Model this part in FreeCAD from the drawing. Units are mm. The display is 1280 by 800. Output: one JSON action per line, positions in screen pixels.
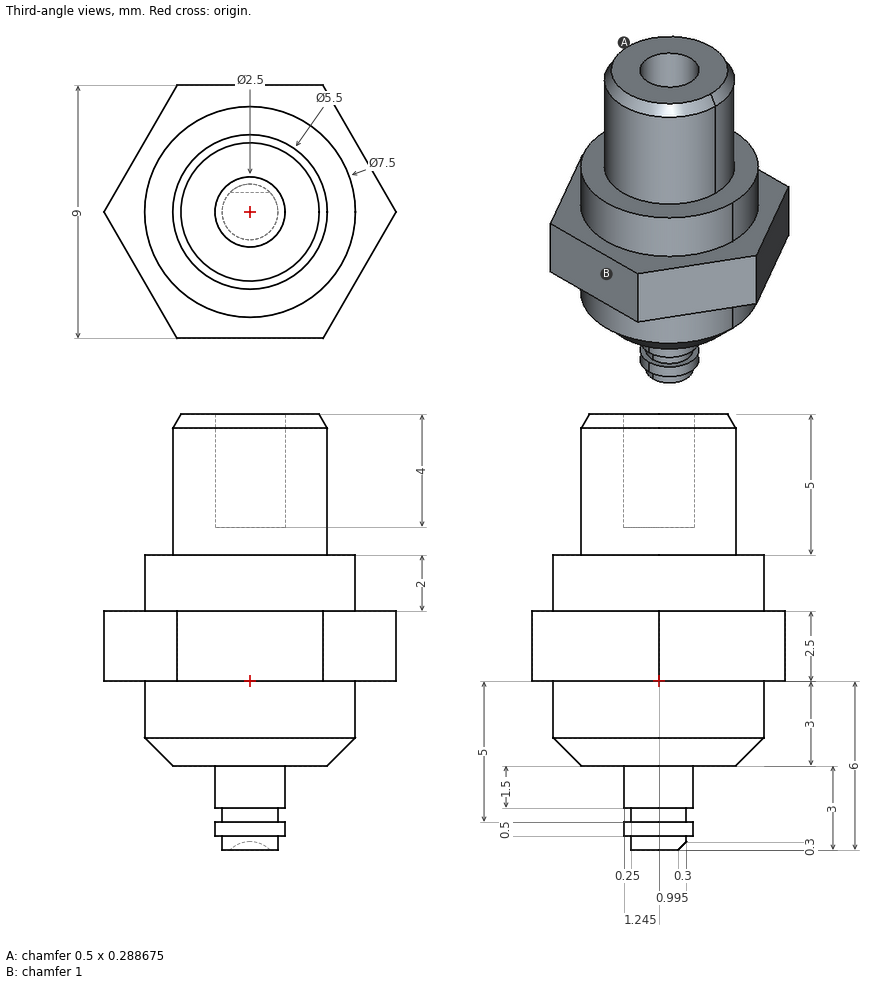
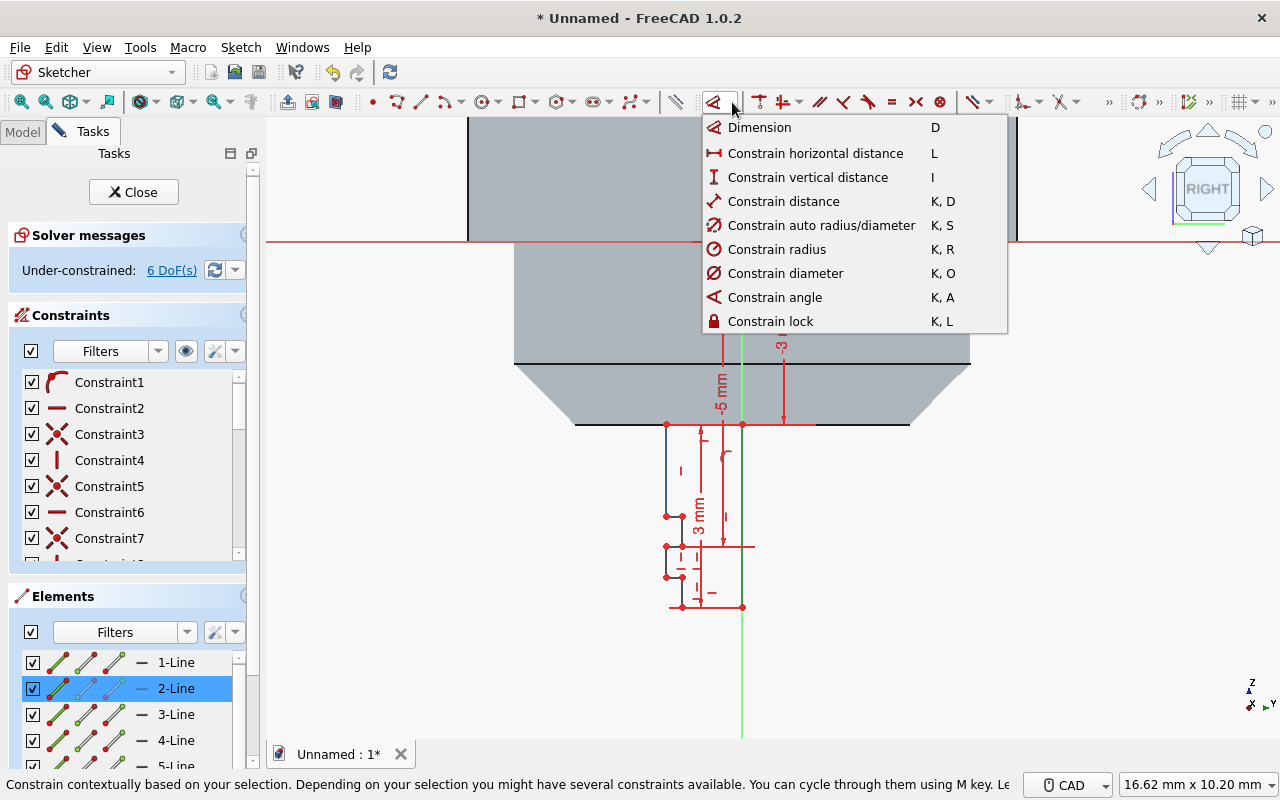
{"action": "left_click", "coordinate": [855, 177]}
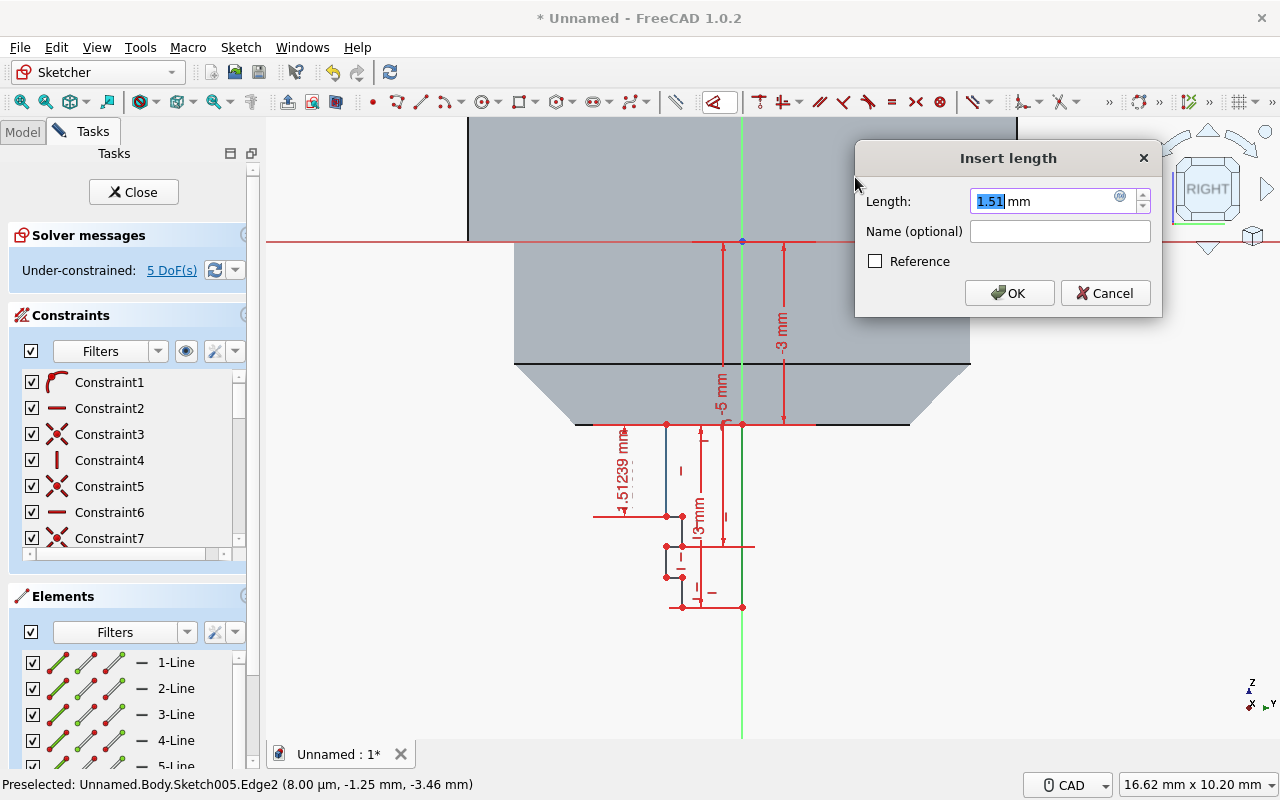
{"action": "type", "text": "1.5"}
{"action": "key", "text": "Return"}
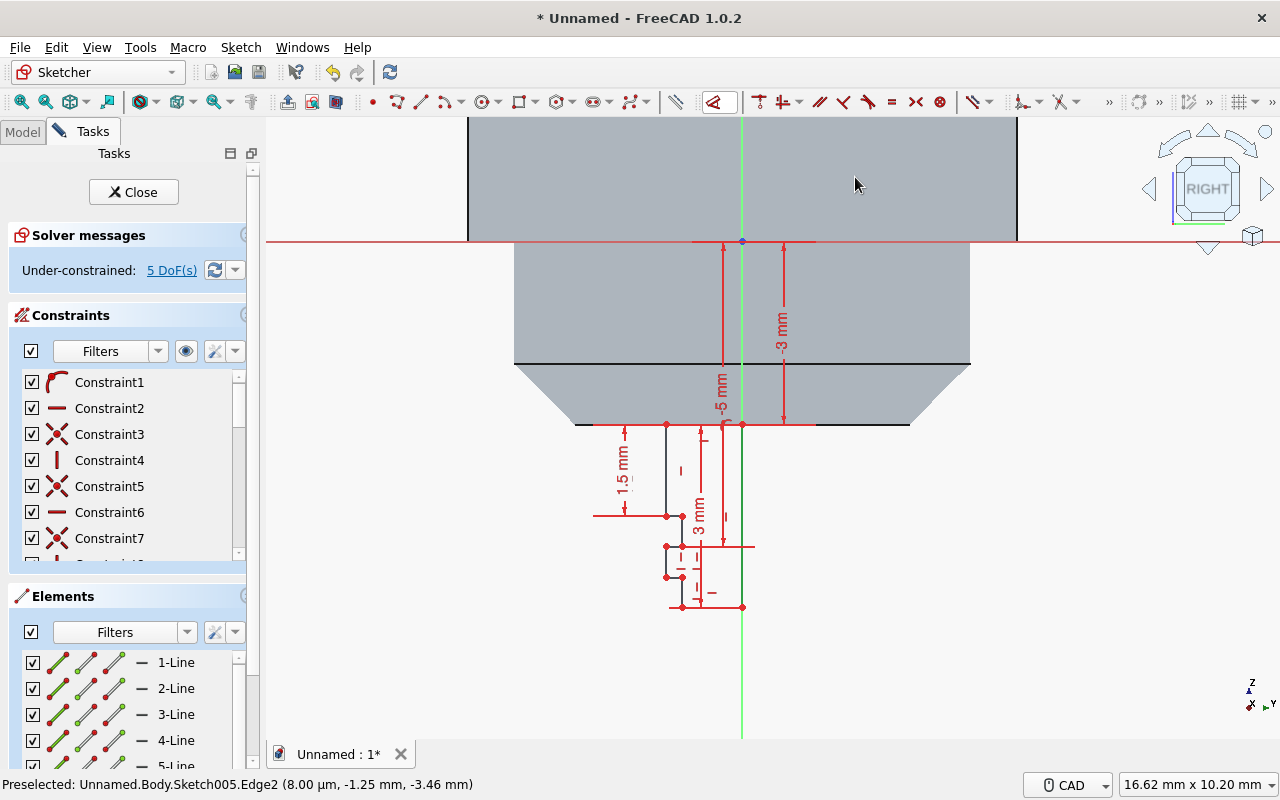
{"action": "scroll", "coordinate": [666, 556], "scroll_direction": "up", "scroll_amount": 2}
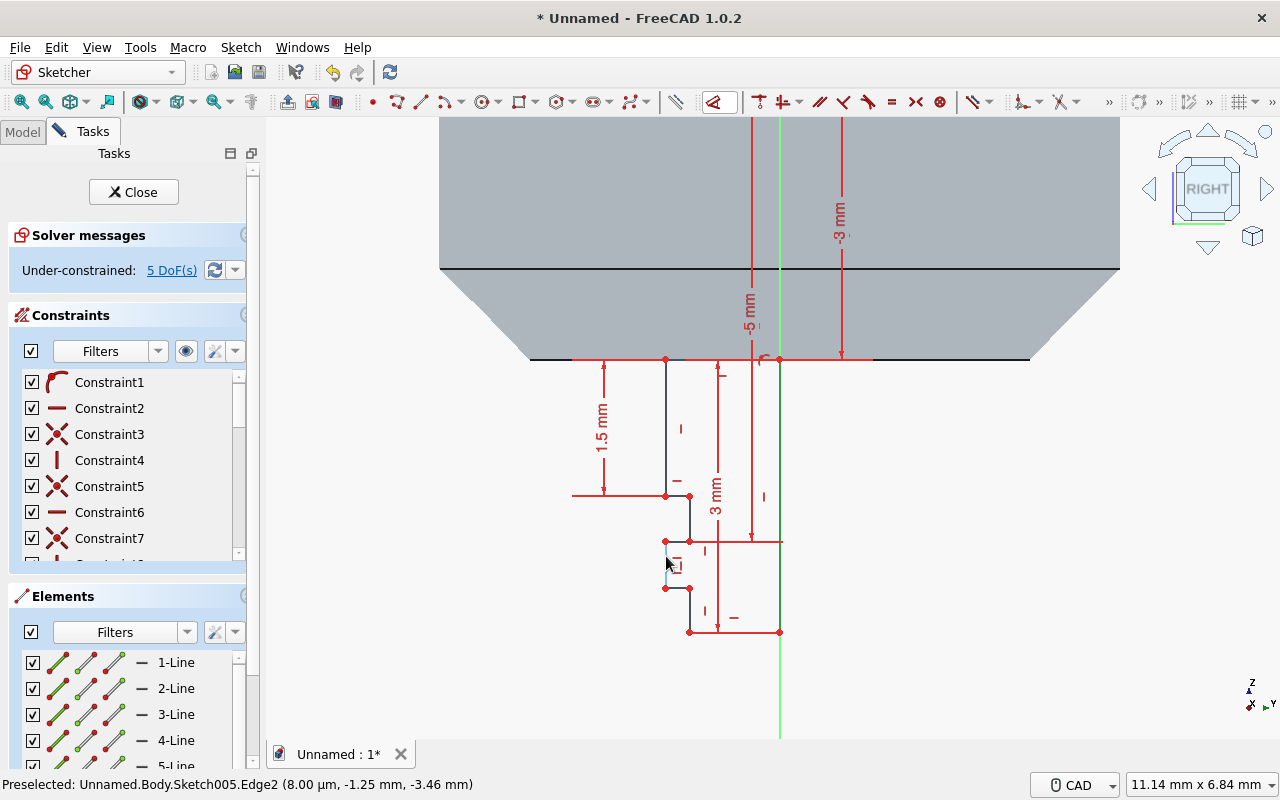
{"action": "left_click", "coordinate": [666, 556]}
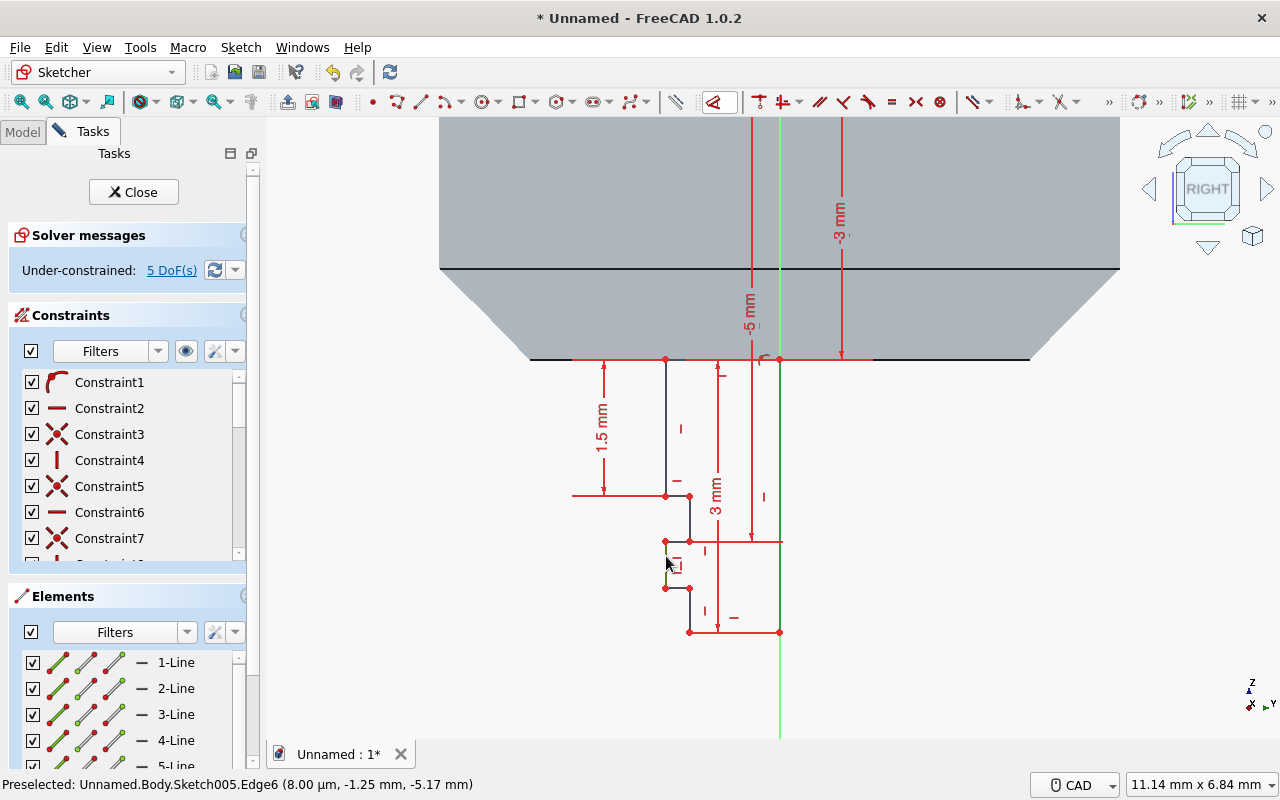
{"action": "key", "text": "i"}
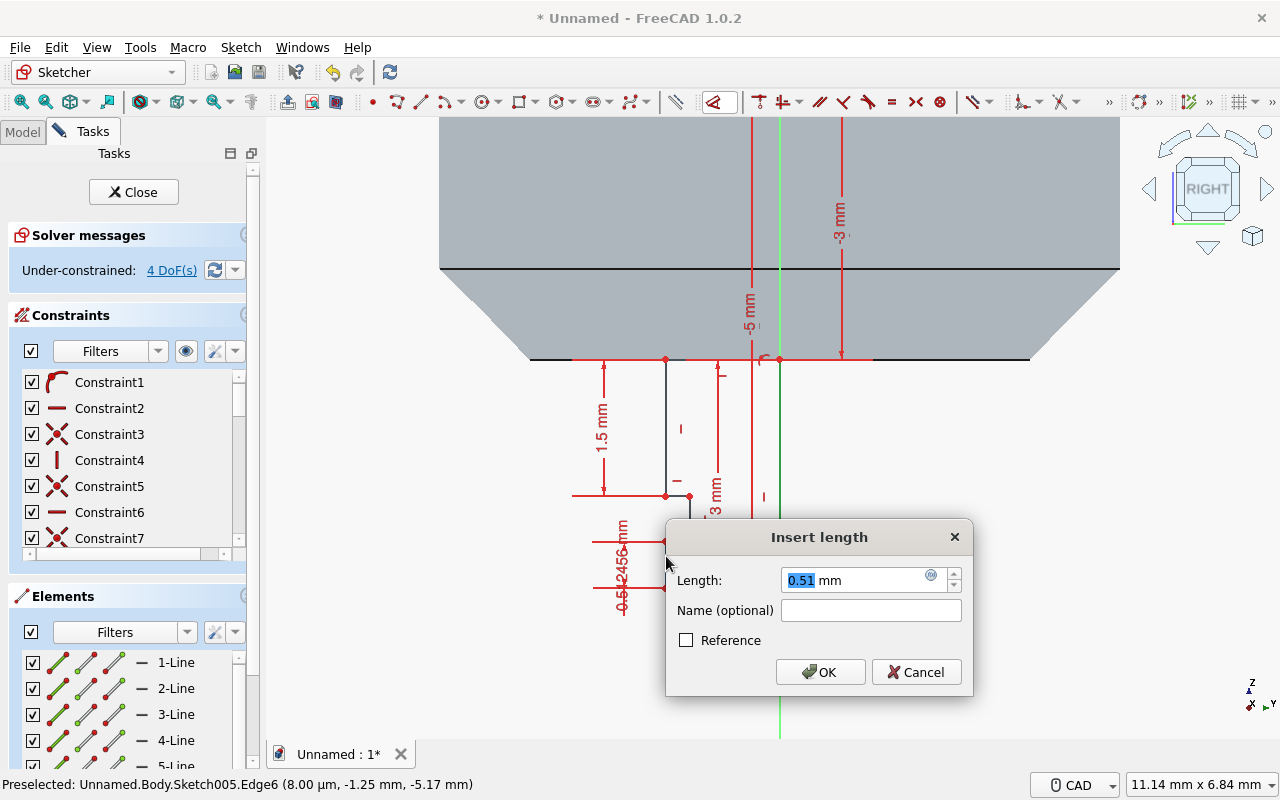
{"action": "type", "text": "0.5"}
{"action": "key", "text": "Return"}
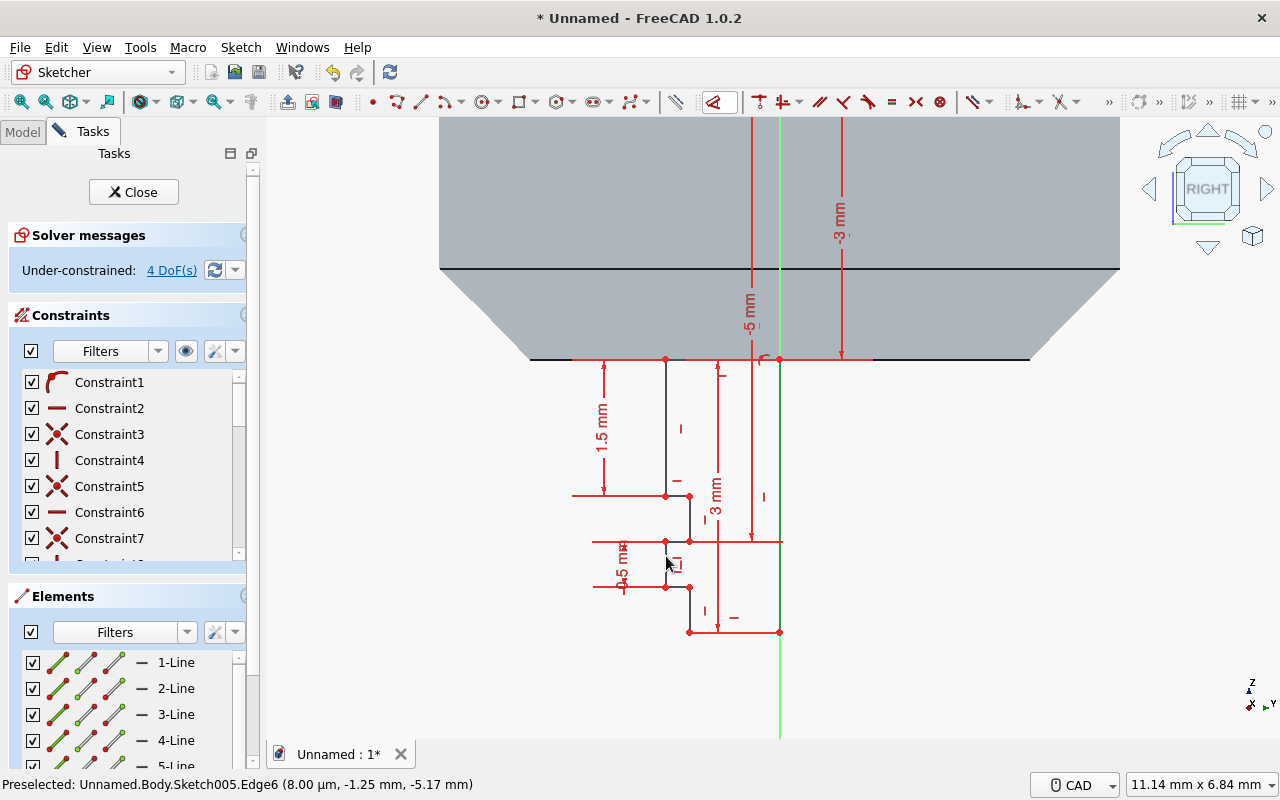
{"action": "scroll", "coordinate": [675, 496], "scroll_direction": "up", "scroll_amount": 3}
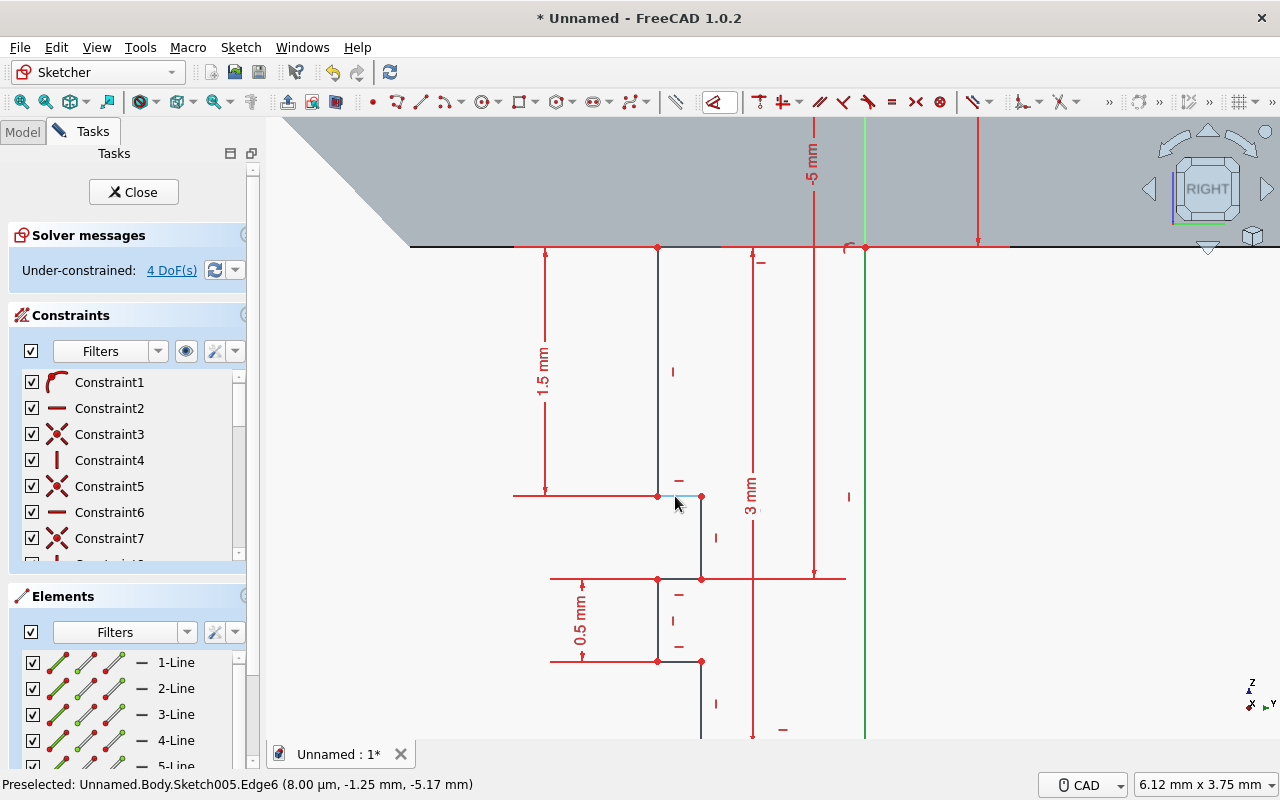
{"action": "left_click", "coordinate": [675, 496]}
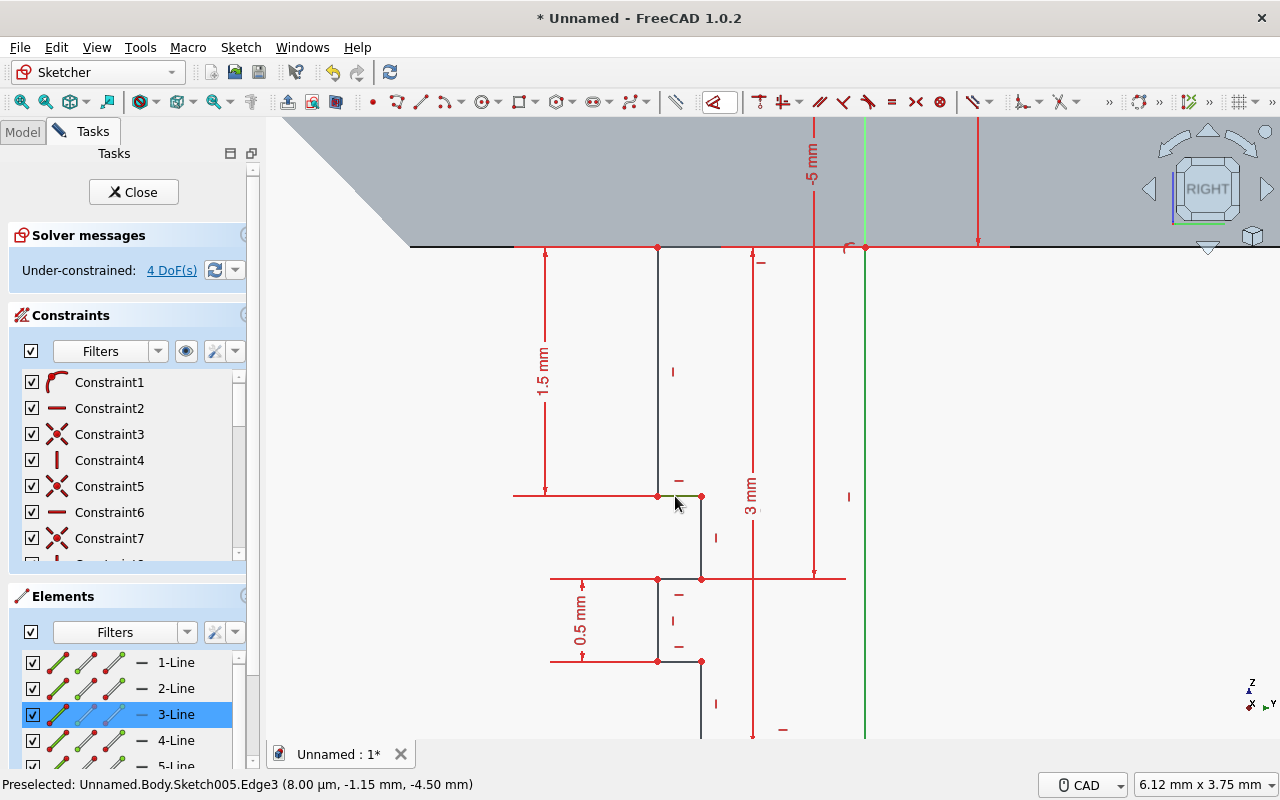
{"action": "left_click", "coordinate": [732, 102]}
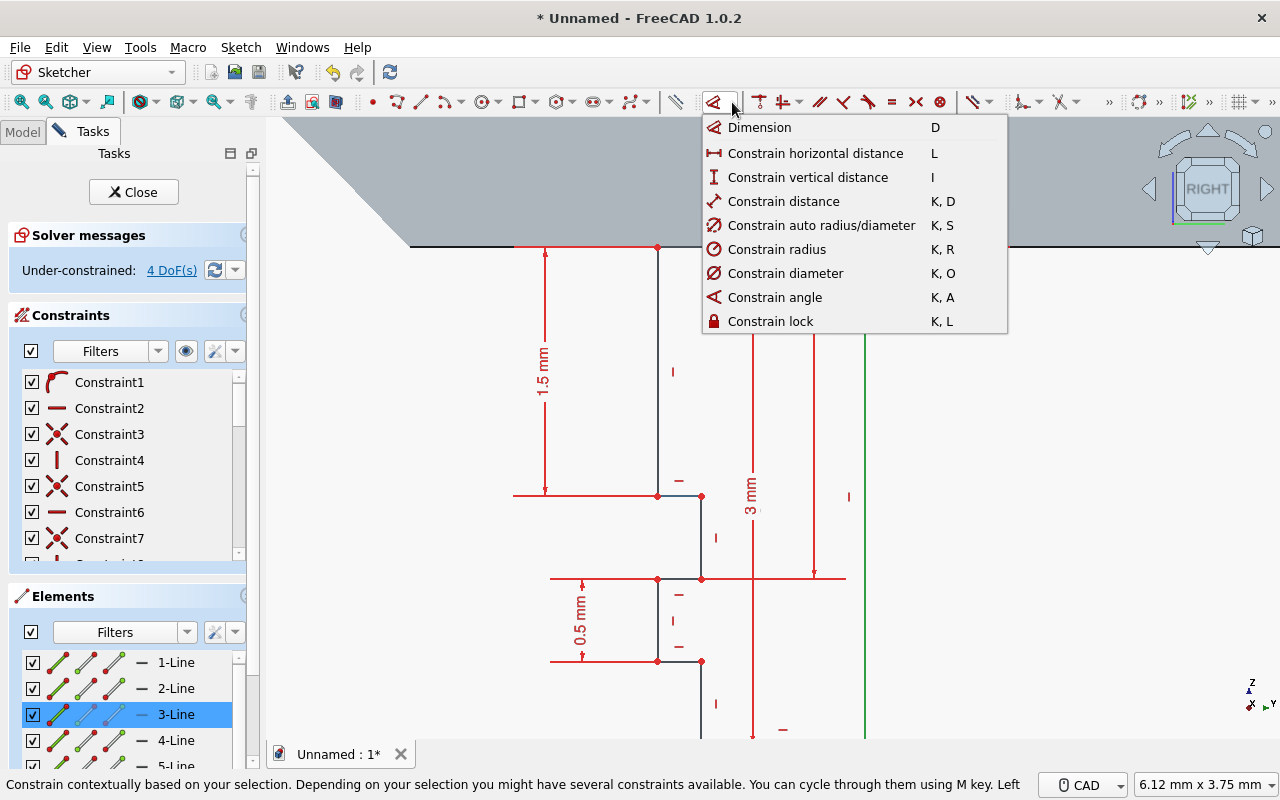
{"action": "left_click", "coordinate": [855, 153]}